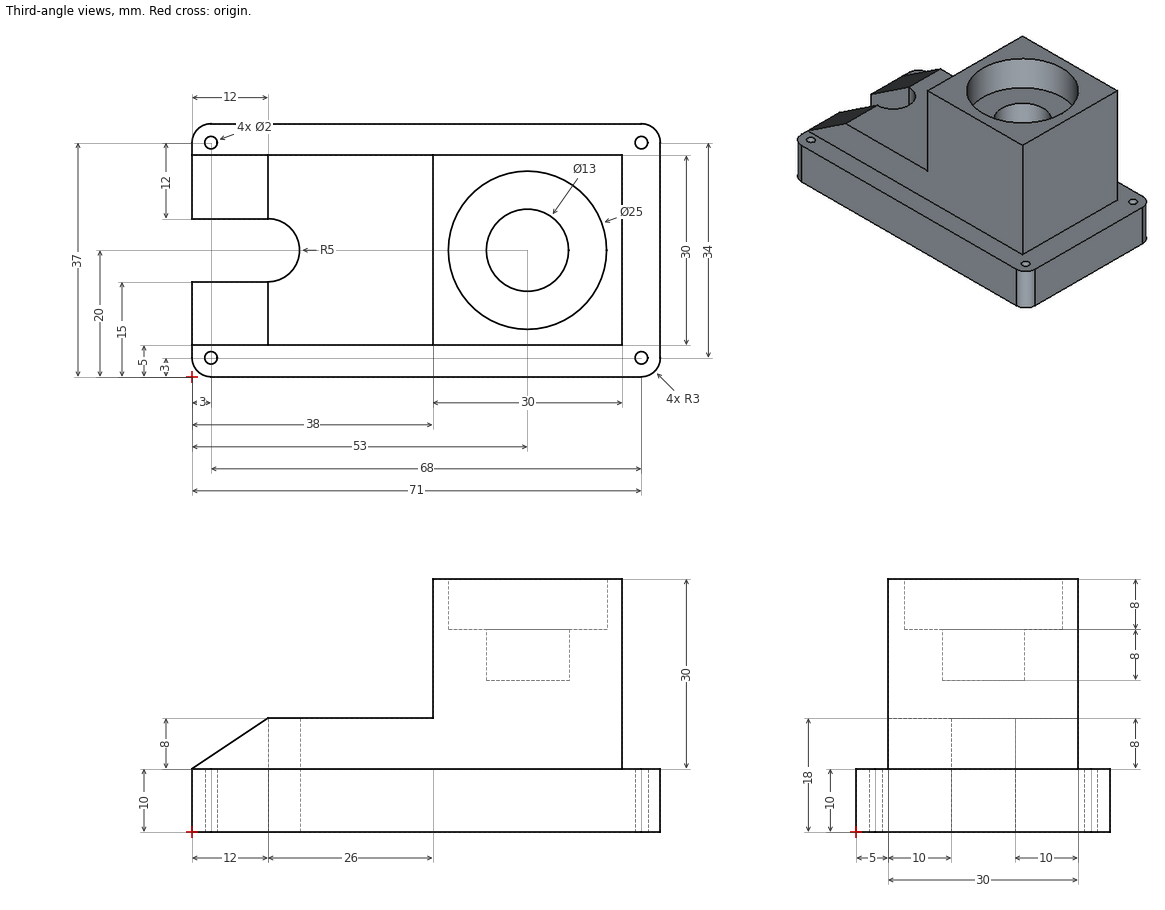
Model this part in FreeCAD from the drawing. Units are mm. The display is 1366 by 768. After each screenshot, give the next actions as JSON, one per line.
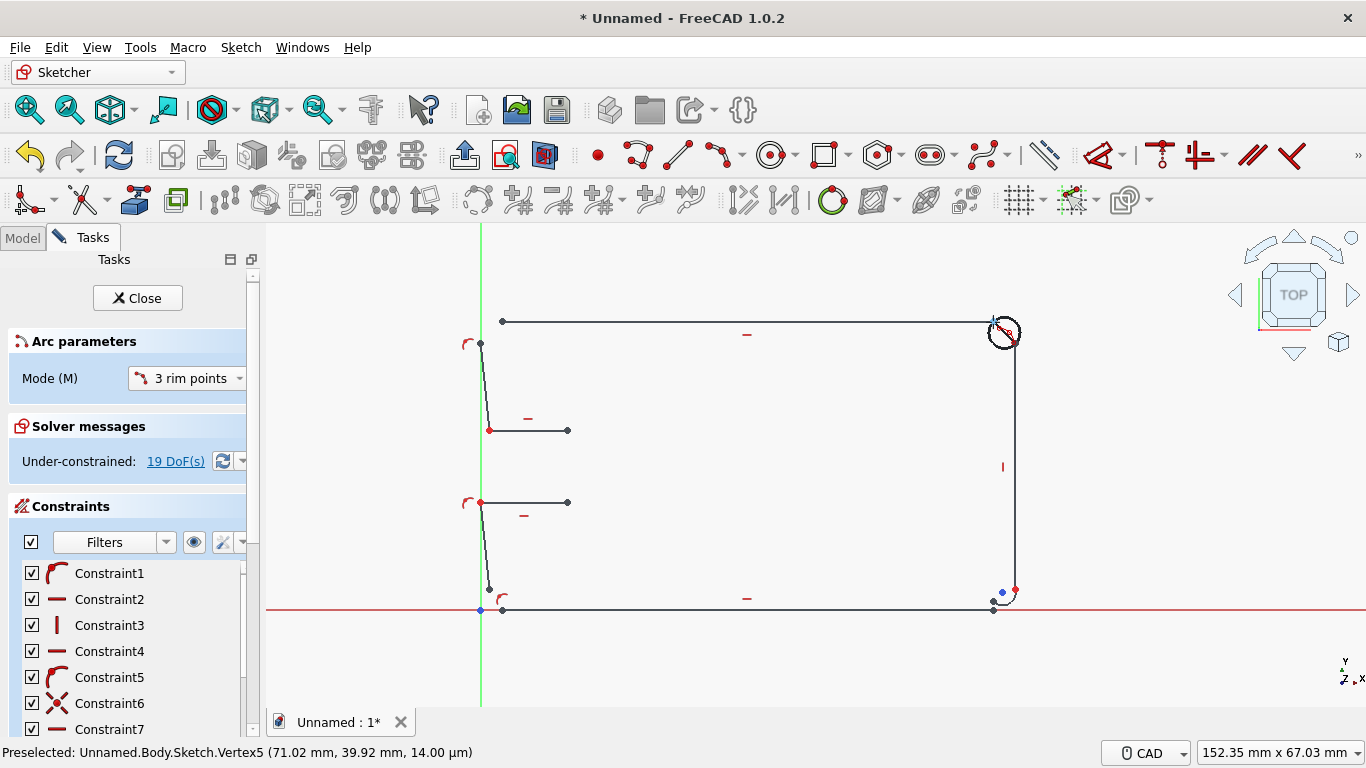
{"action": "scroll", "coordinate": [1009, 328], "scroll_direction": "up", "scroll_amount": 5}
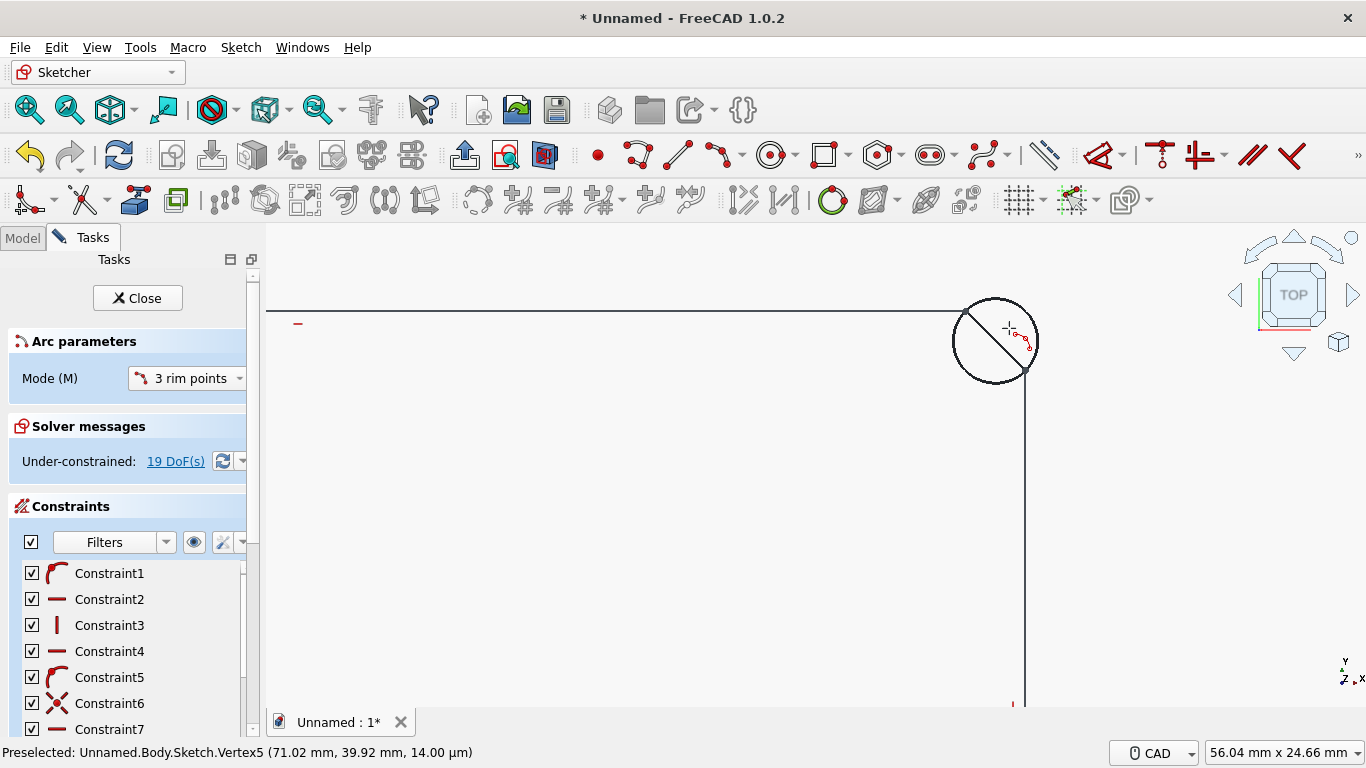
{"action": "left_click", "coordinate": [1007, 327]}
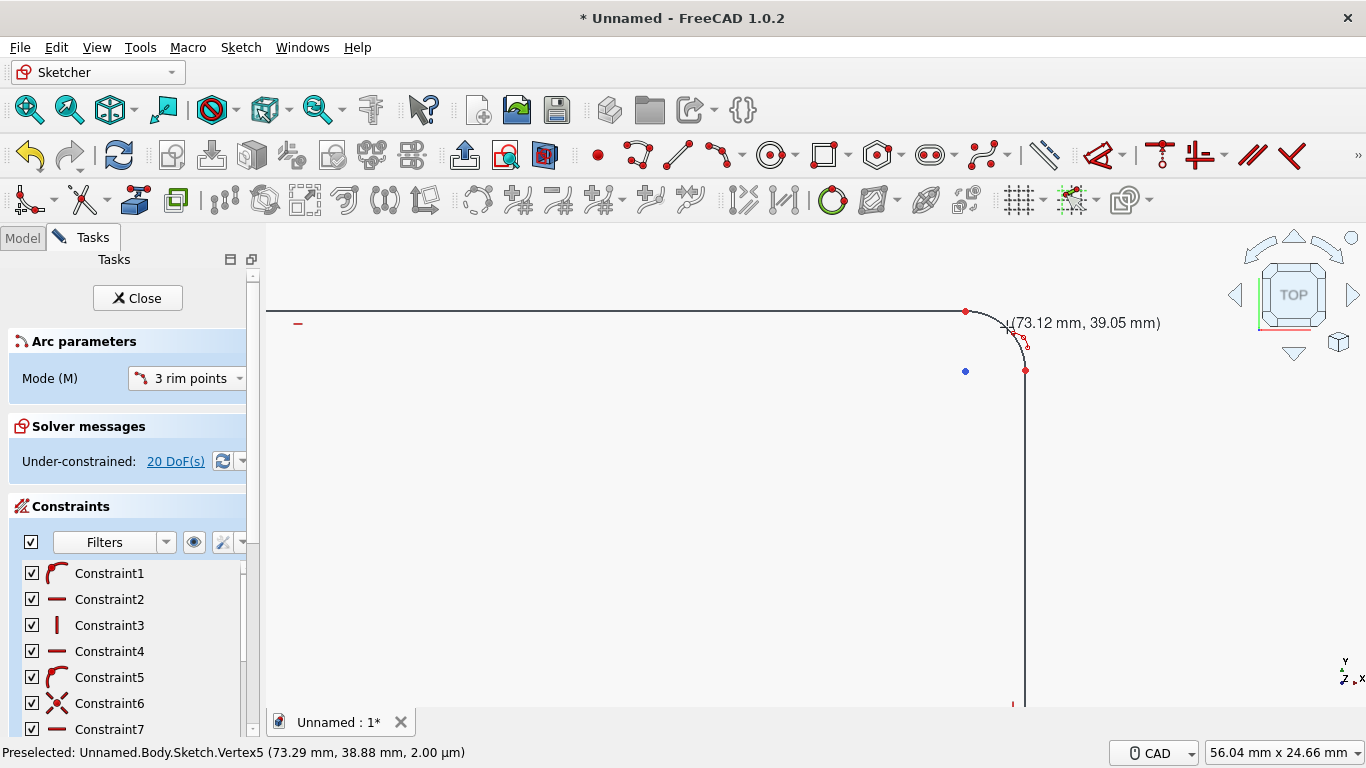
{"action": "scroll", "coordinate": [1009, 327], "scroll_direction": "down", "scroll_amount": 5}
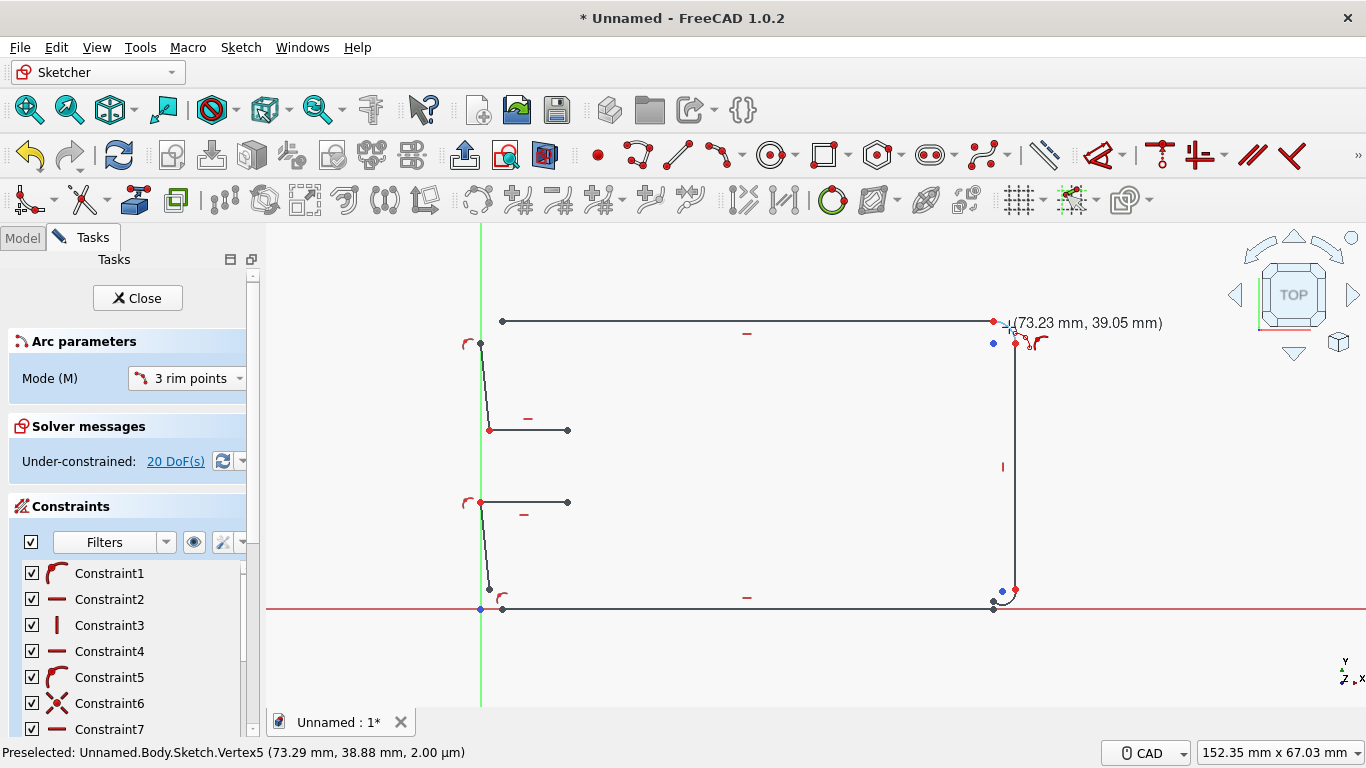
{"action": "left_click", "coordinate": [502, 321]}
{"action": "left_click", "coordinate": [481, 343]}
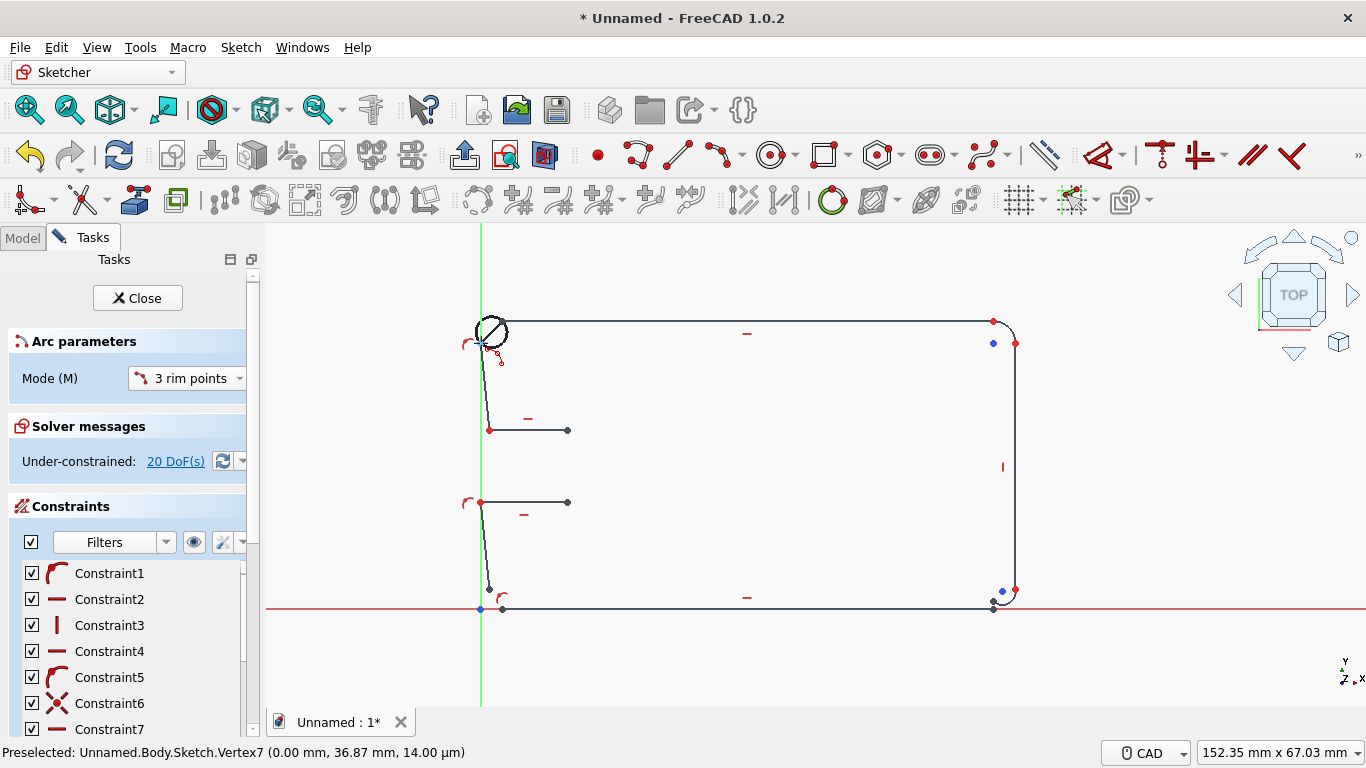
{"action": "scroll", "coordinate": [487, 327], "scroll_direction": "up", "scroll_amount": 5}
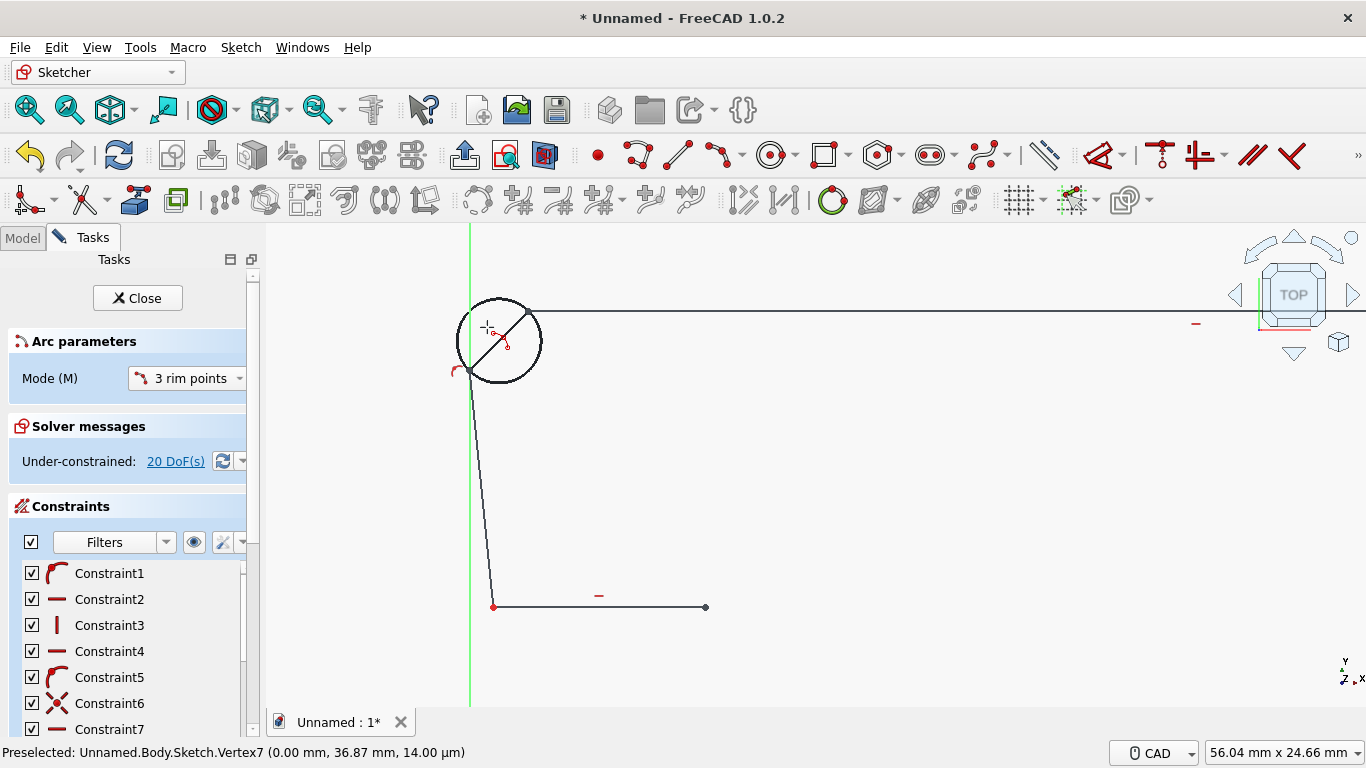
{"action": "left_click", "coordinate": [487, 327]}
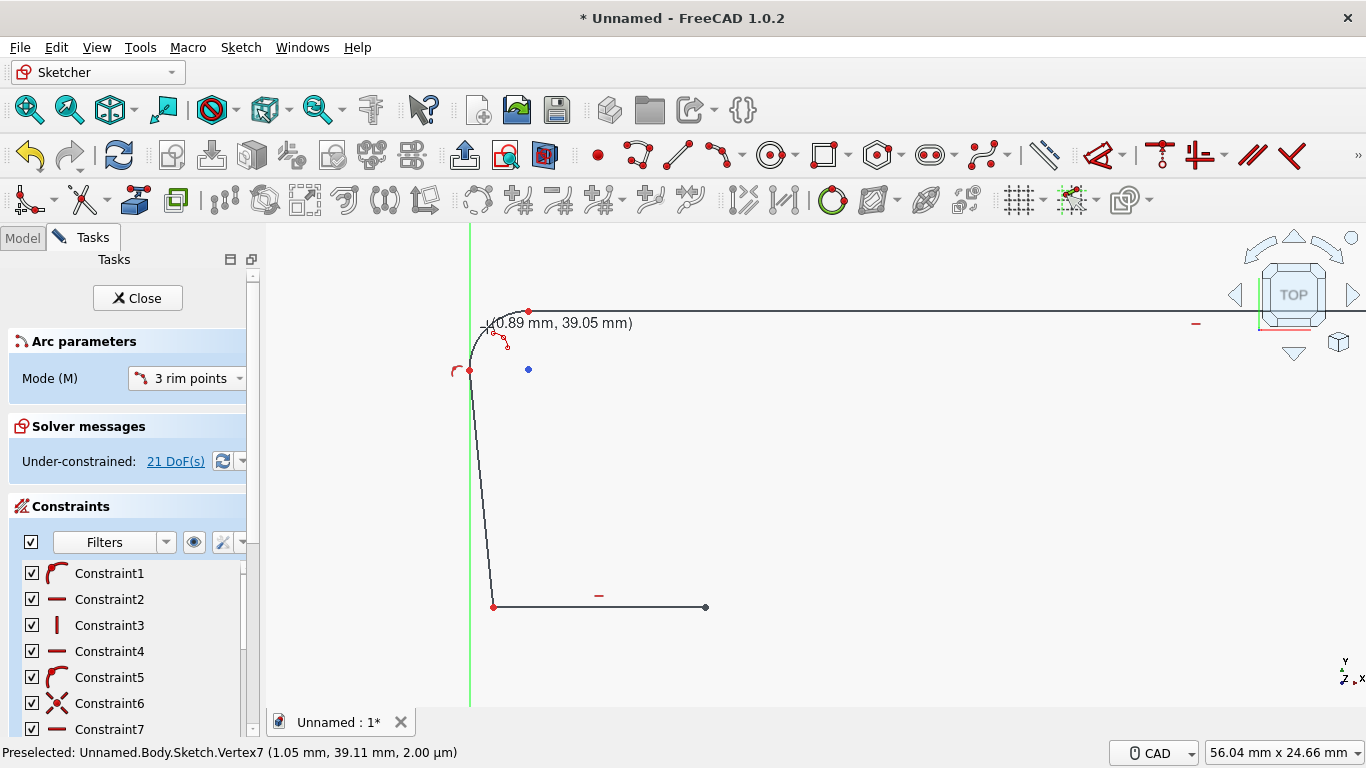
{"action": "left_click", "coordinate": [705, 607]}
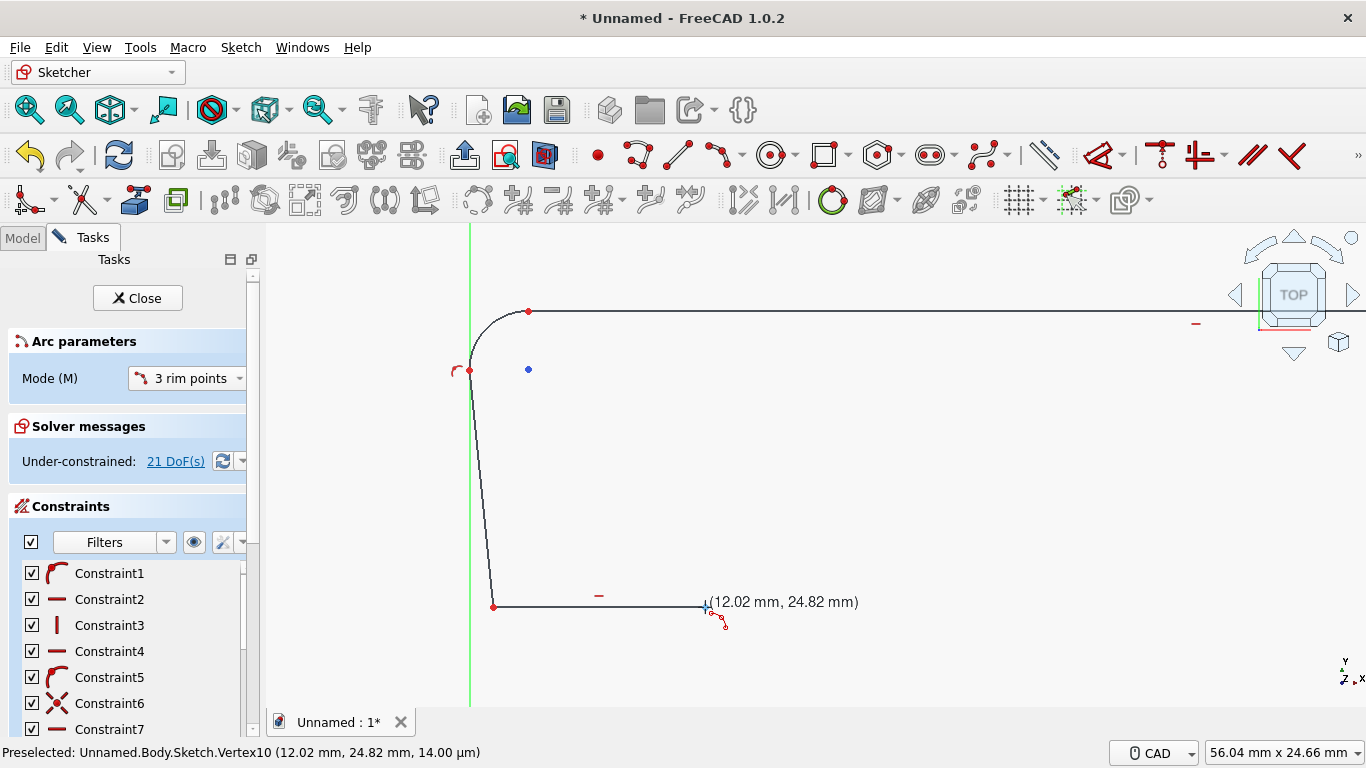
{"action": "scroll", "coordinate": [487, 327], "scroll_direction": "down", "scroll_amount": 5}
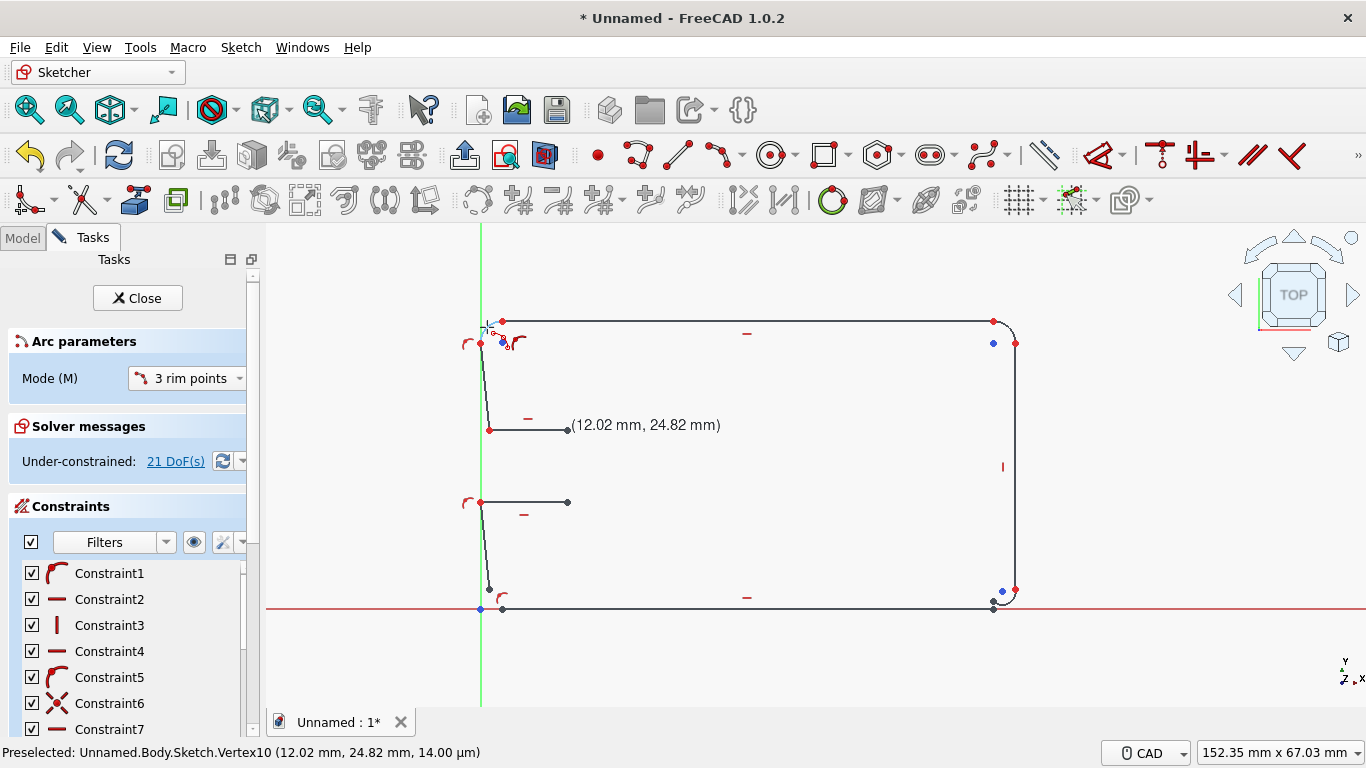
{"action": "left_click", "coordinate": [567, 502]}
{"action": "left_click", "coordinate": [603, 465]}